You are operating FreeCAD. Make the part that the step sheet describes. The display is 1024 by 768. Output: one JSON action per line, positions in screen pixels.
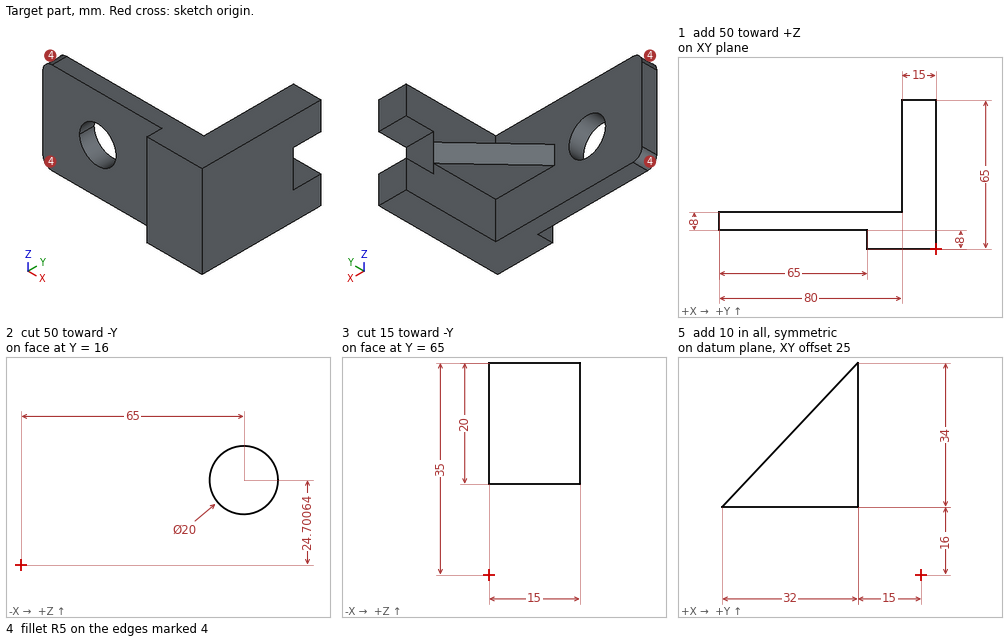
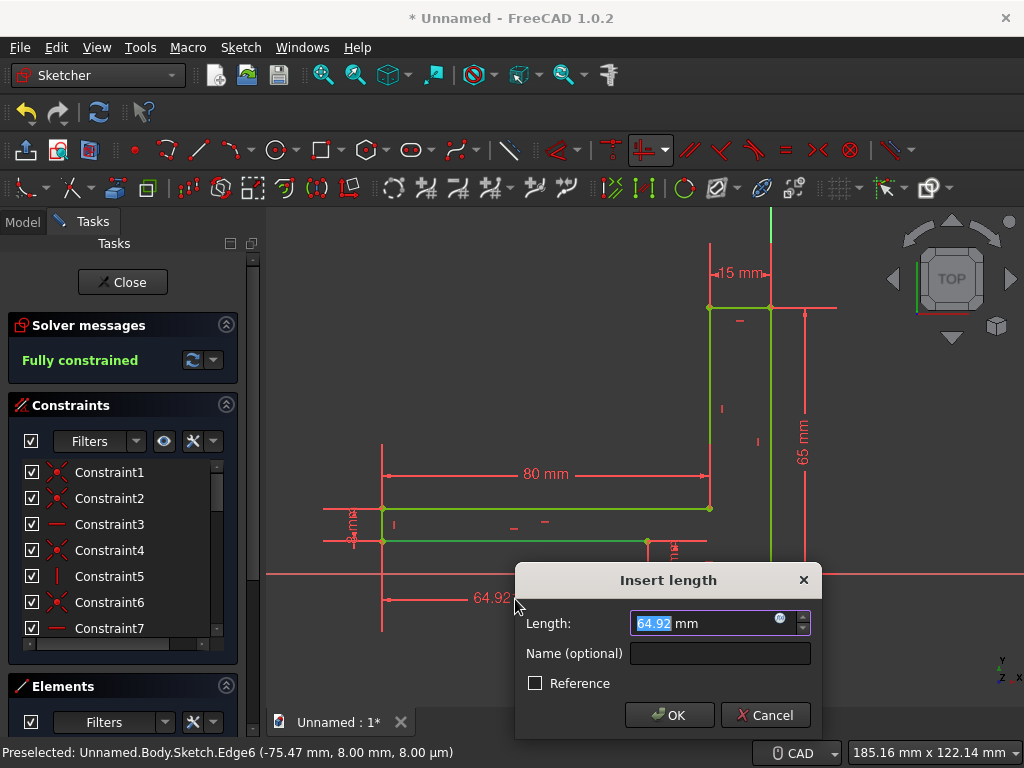
{"action": "type", "text": "65"}
{"action": "key", "text": "Return"}
{"action": "key", "text": "Escape"}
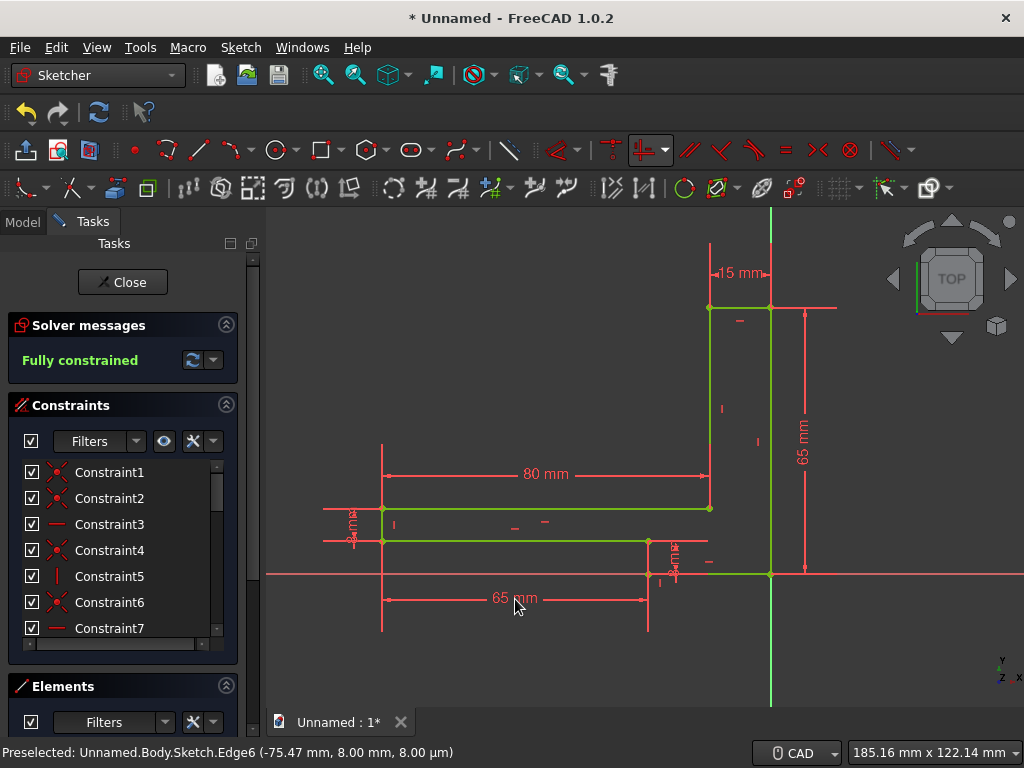
{"action": "left_click", "coordinate": [123, 282]}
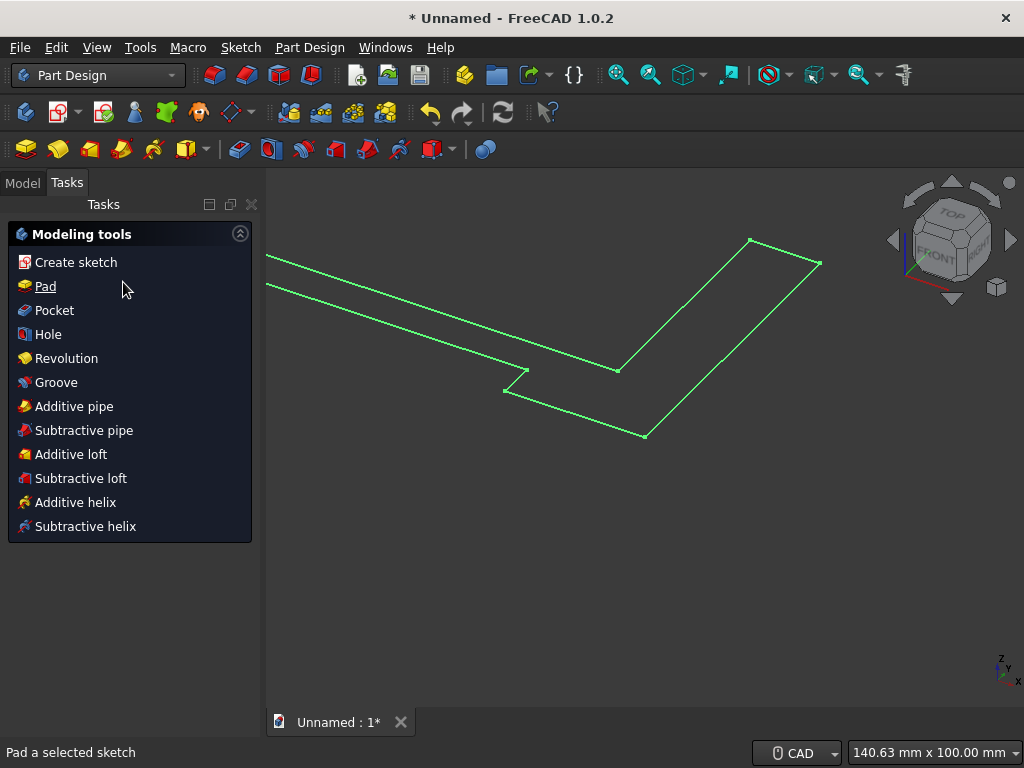
{"action": "left_click", "coordinate": [26, 150]}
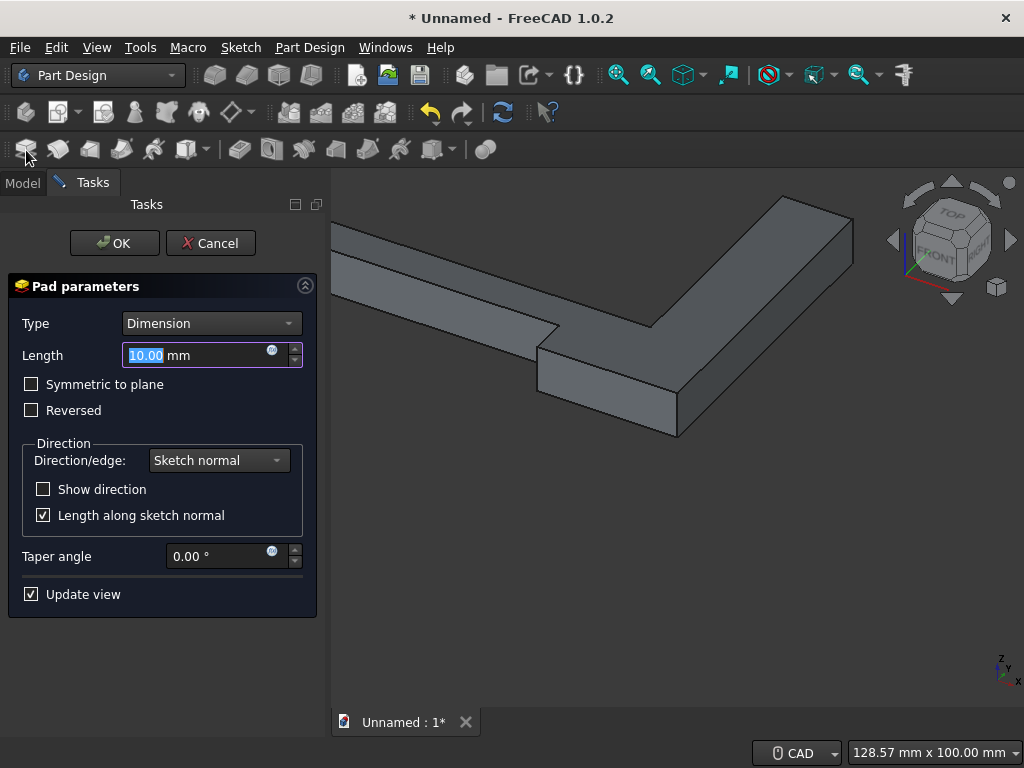
{"action": "type", "text": "50"}
{"action": "key", "text": "Tab"}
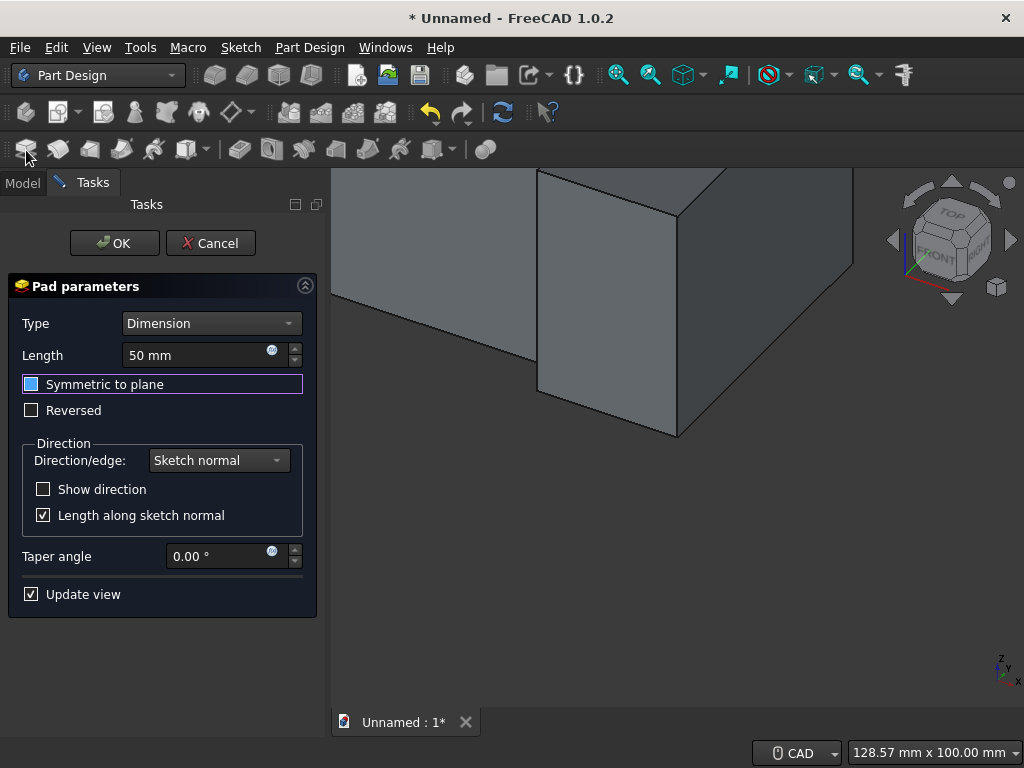
{"action": "left_click", "coordinate": [115, 243]}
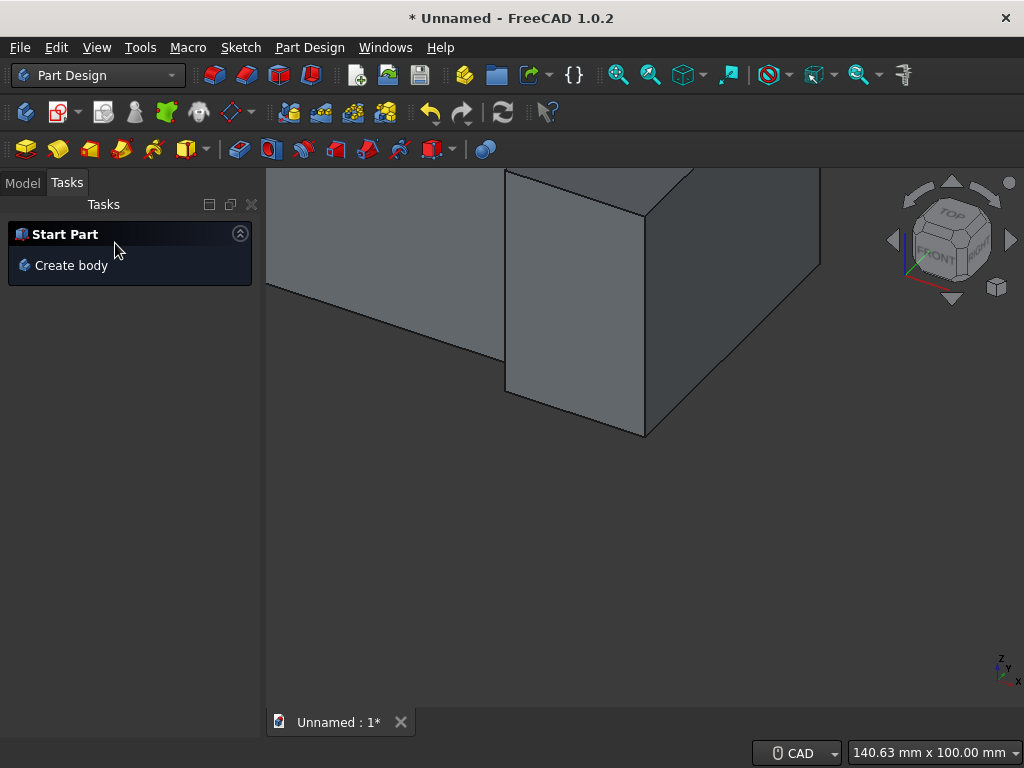
{"action": "left_click", "coordinate": [620, 76]}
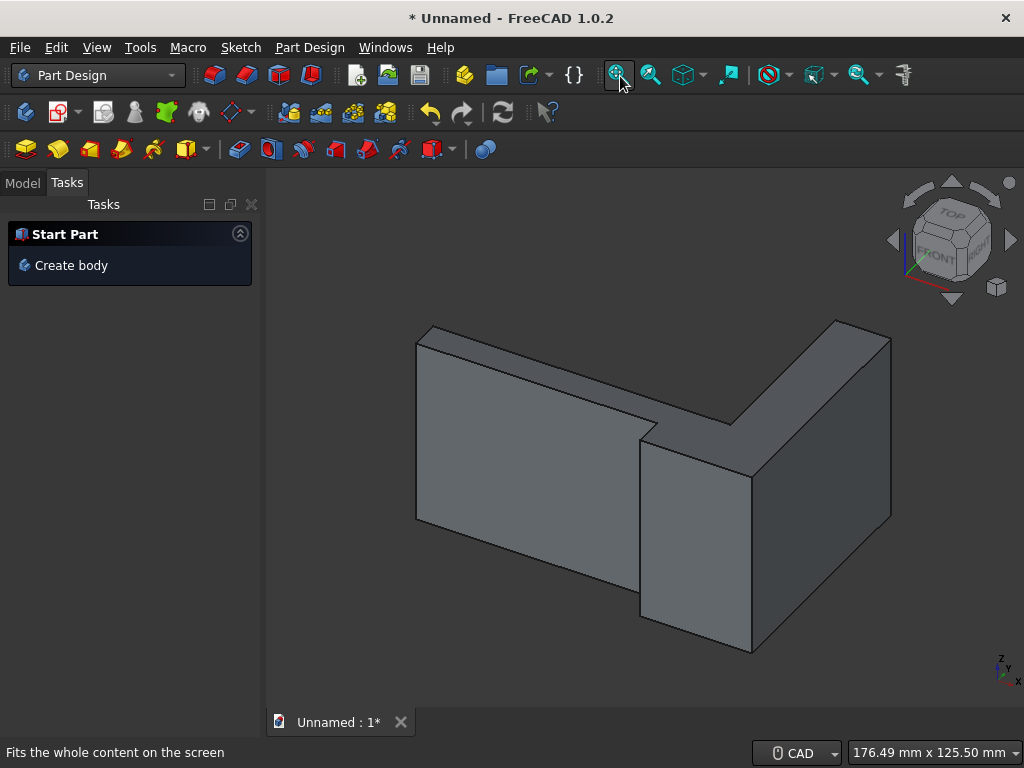
{"action": "key", "text": "4"}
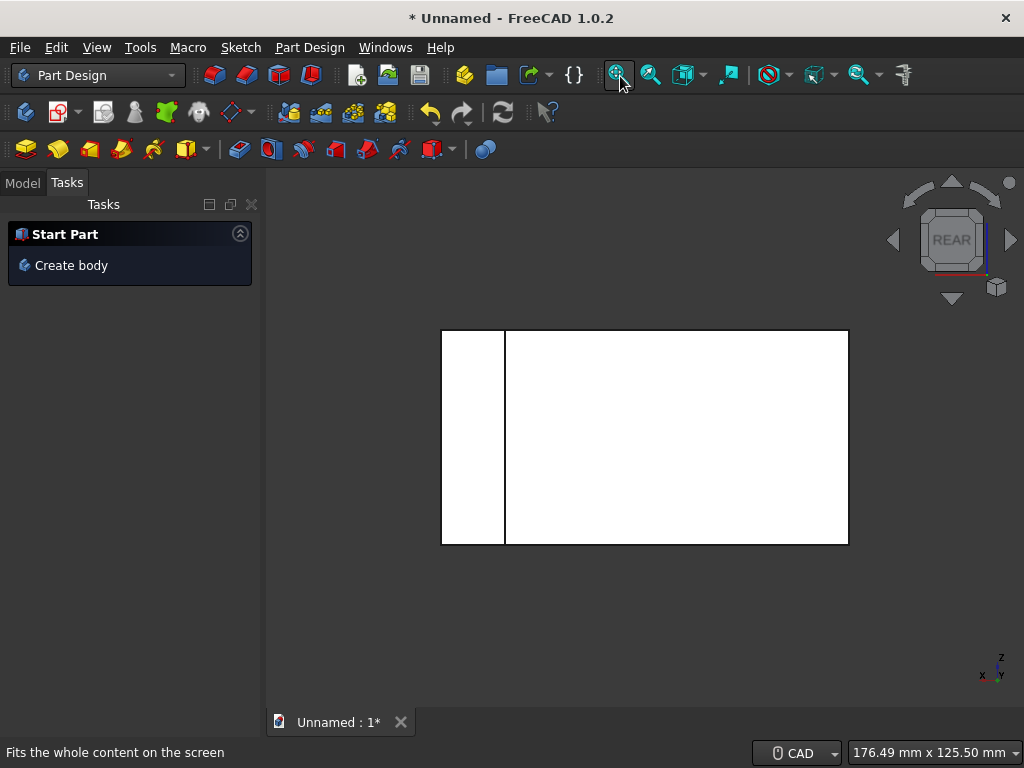
{"action": "left_click", "coordinate": [628, 436]}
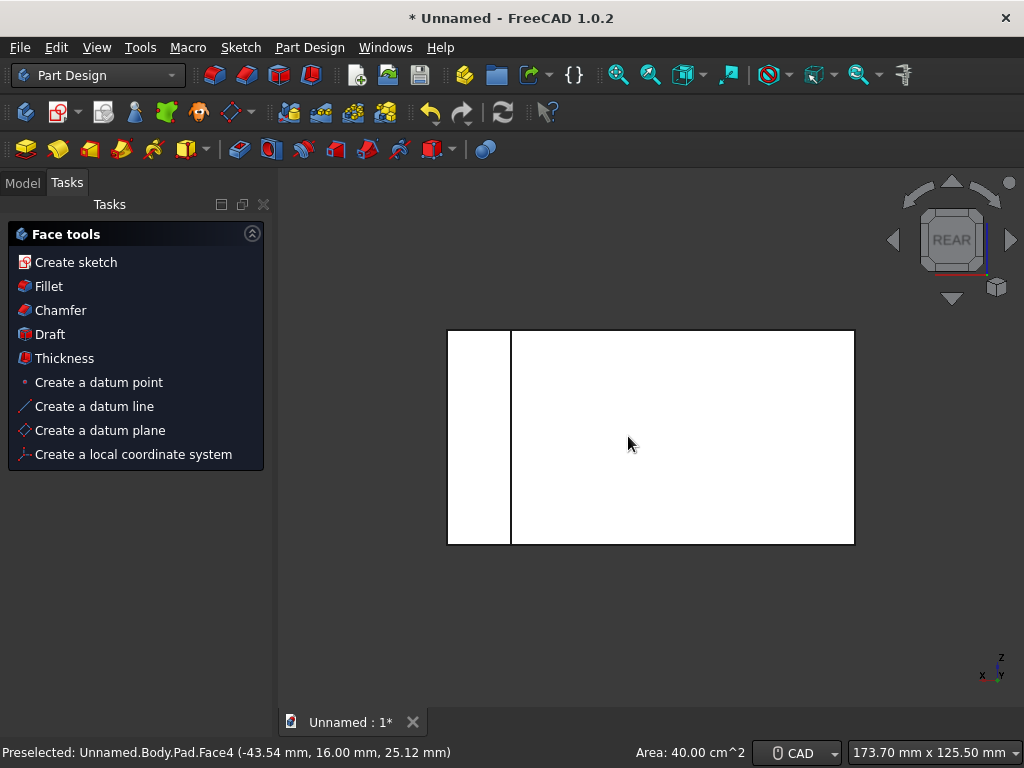
{"action": "left_click", "coordinate": [58, 112]}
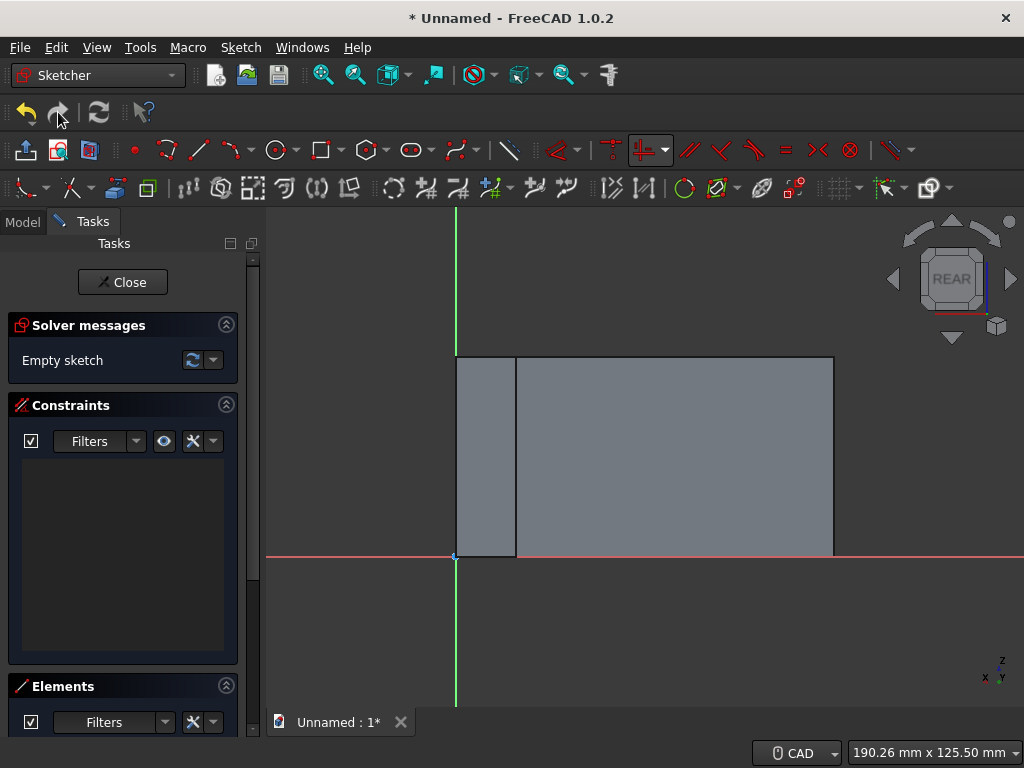
{"action": "left_click", "coordinate": [90, 150]}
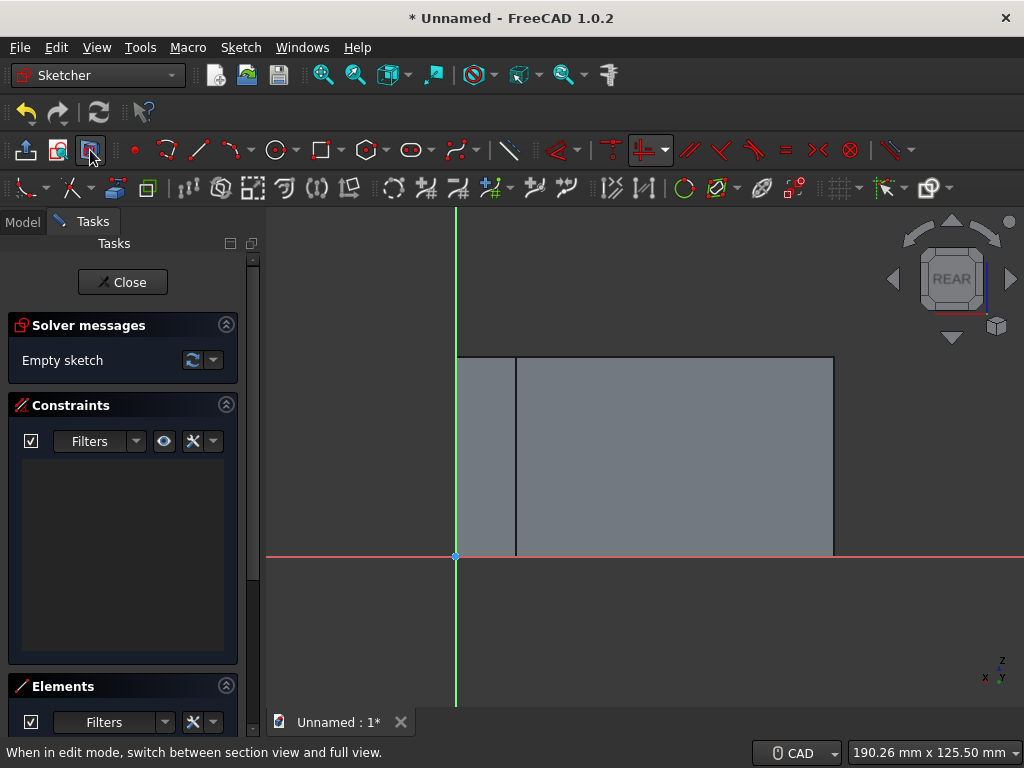
{"action": "scroll", "coordinate": [760, 459], "scroll_direction": "up", "scroll_amount": 7}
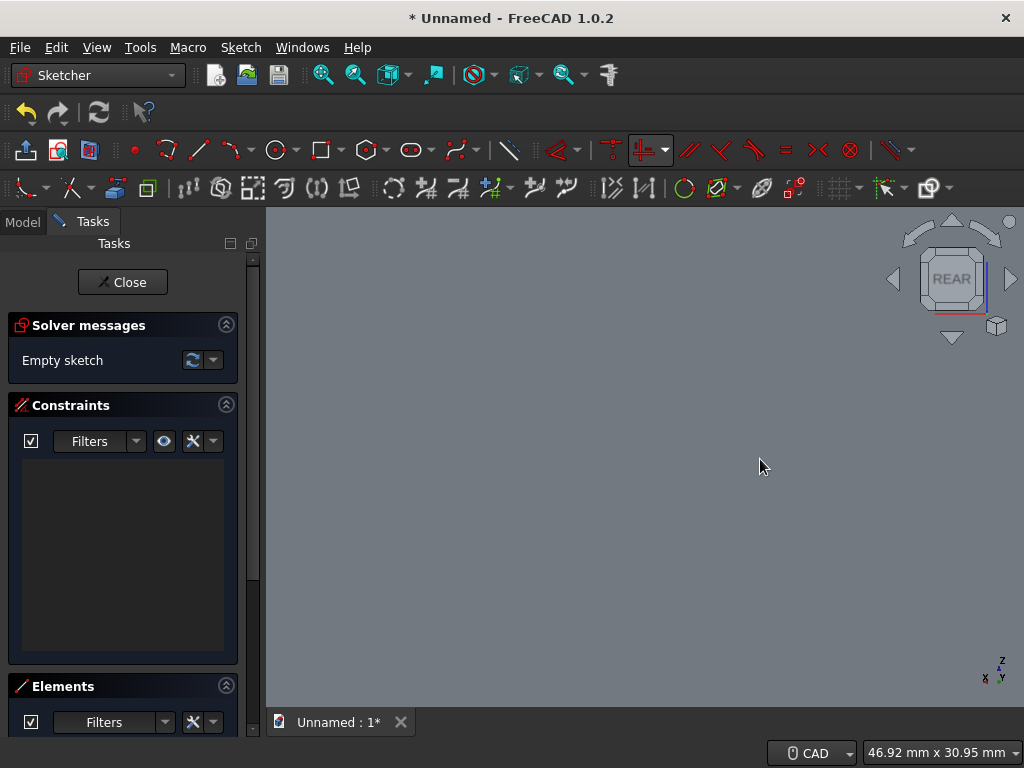
{"action": "left_click", "coordinate": [276, 150]}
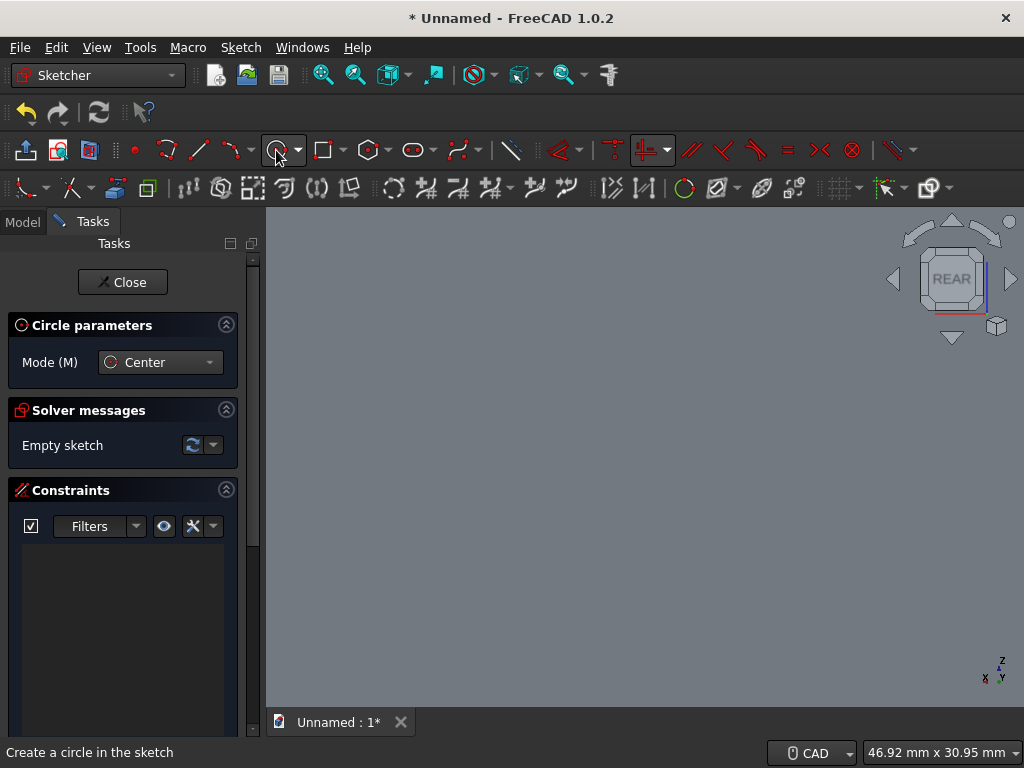
{"action": "left_click", "coordinate": [574, 454]}
{"action": "left_click", "coordinate": [689, 340]}
{"action": "key", "text": "Escape"}